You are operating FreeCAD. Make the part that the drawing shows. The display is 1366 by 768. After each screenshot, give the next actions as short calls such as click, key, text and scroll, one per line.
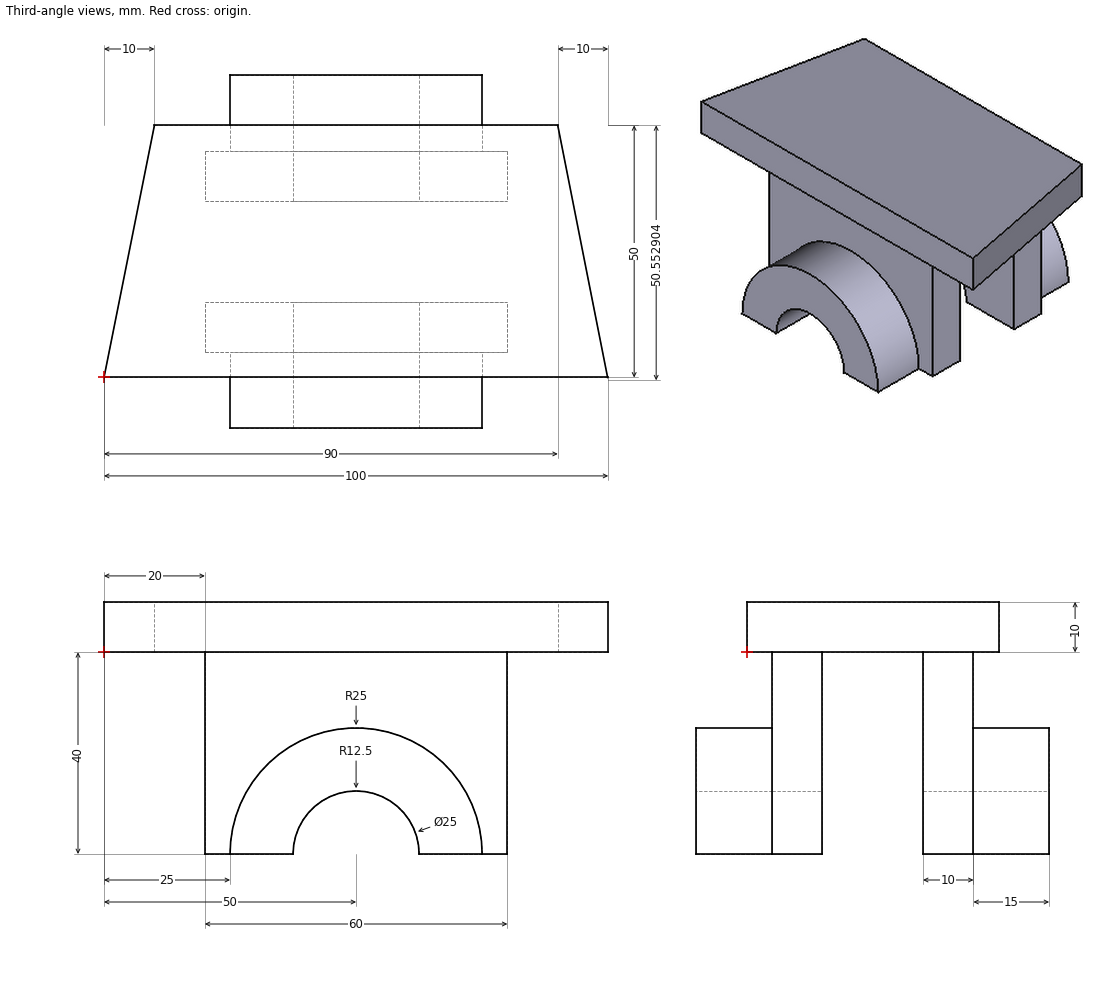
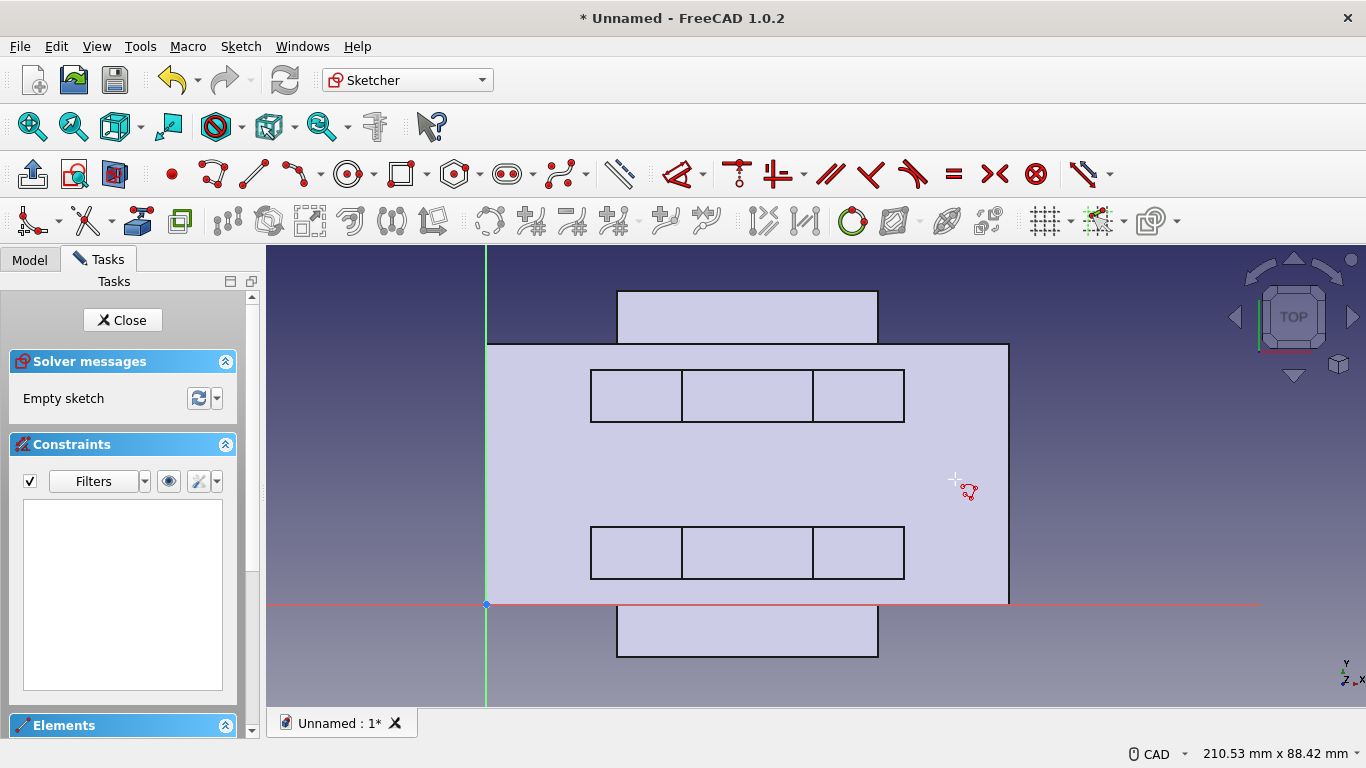
scroll(1009, 608, up, 9)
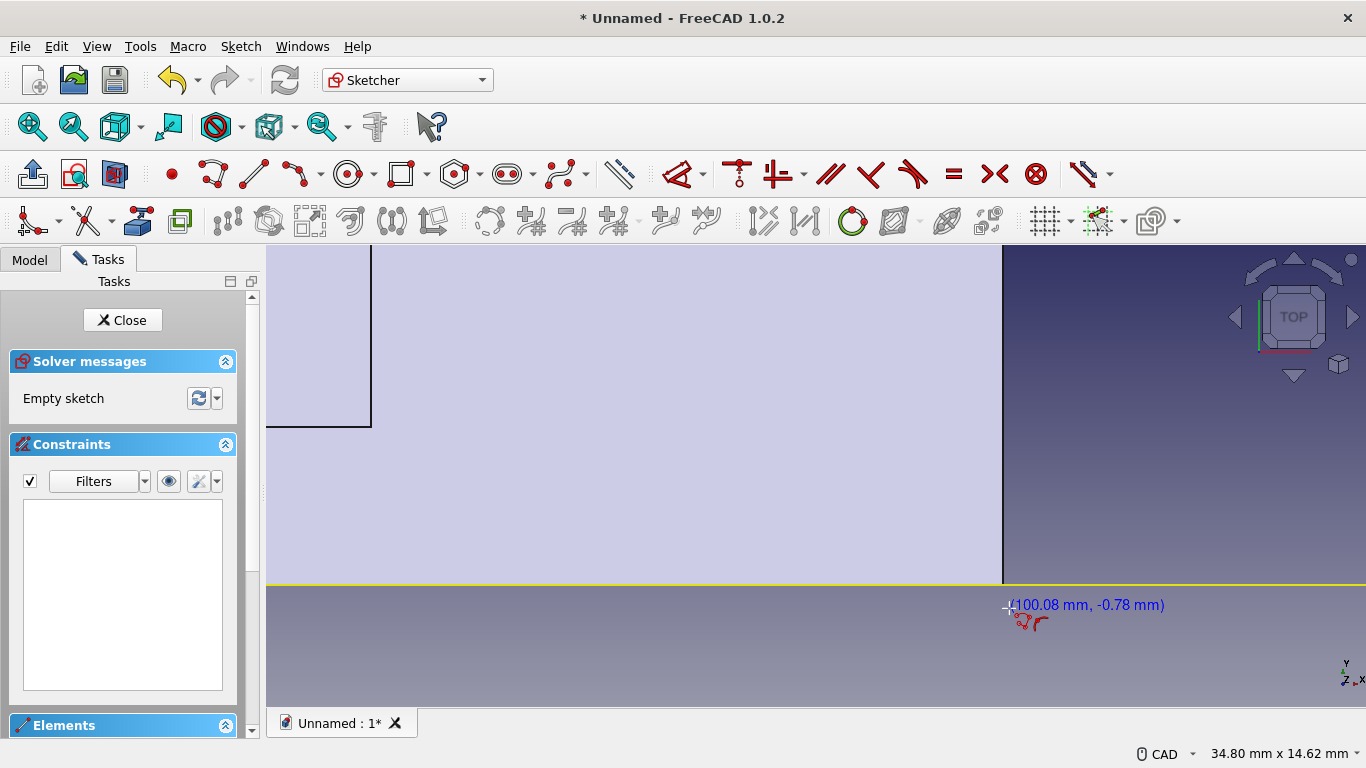
click(1003, 603)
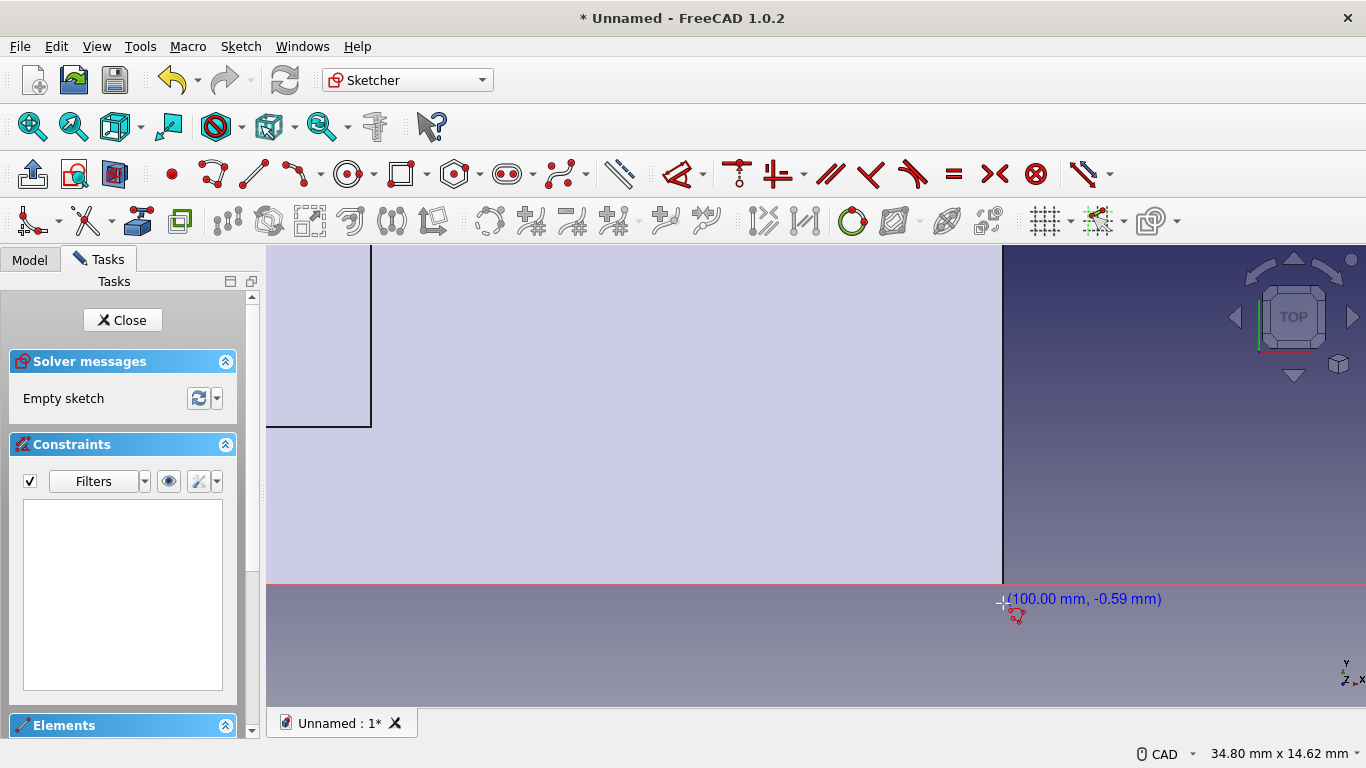
scroll(1010, 609, down, 9)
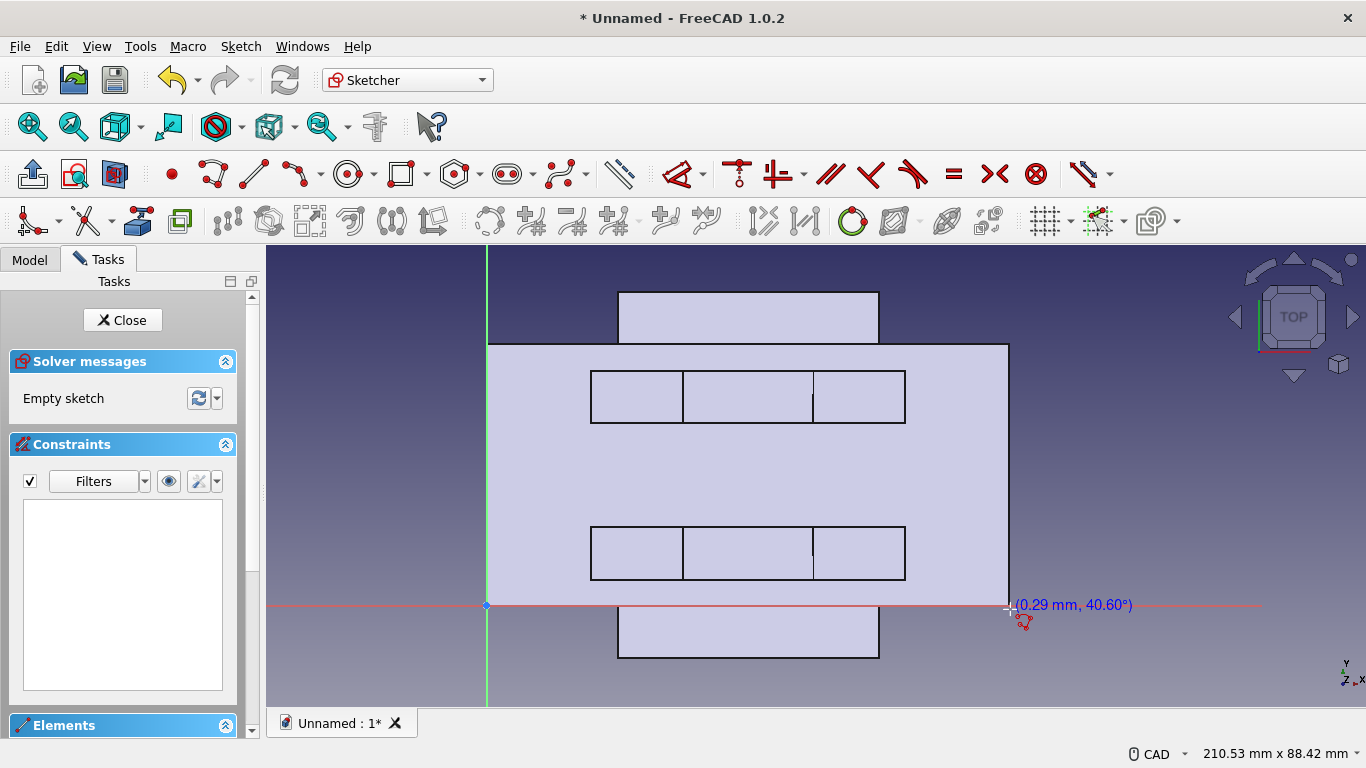
click(957, 344)
click(1009, 344)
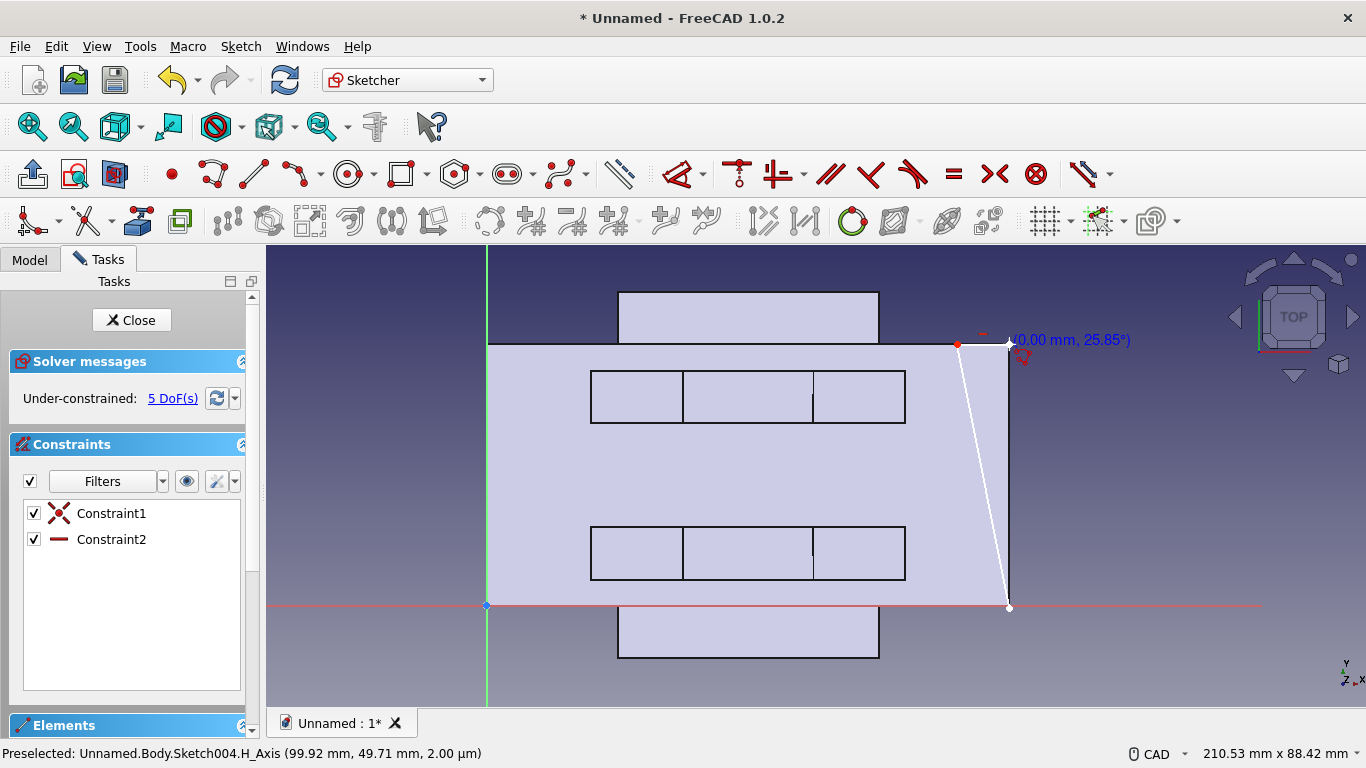
scroll(1009, 609, up, 9)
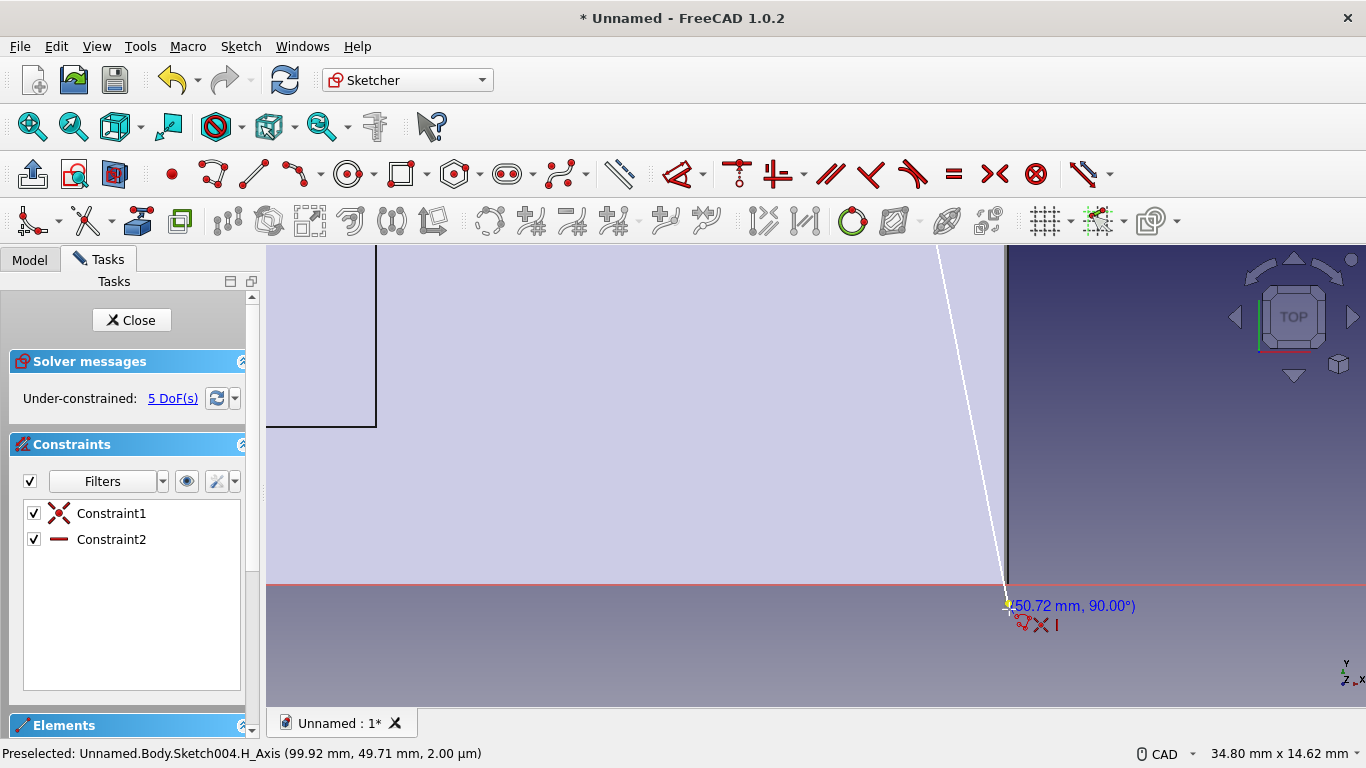
click(1008, 604)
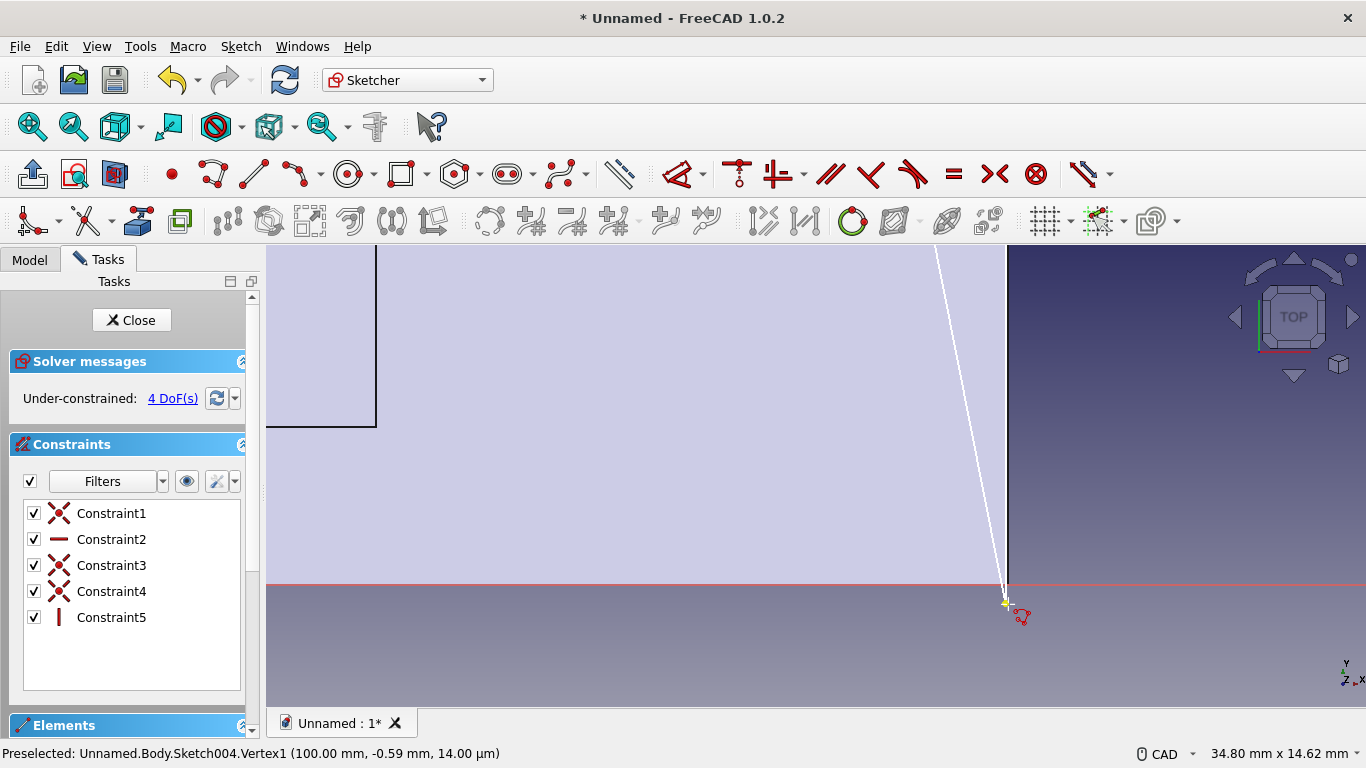
scroll(1009, 609, down, 9)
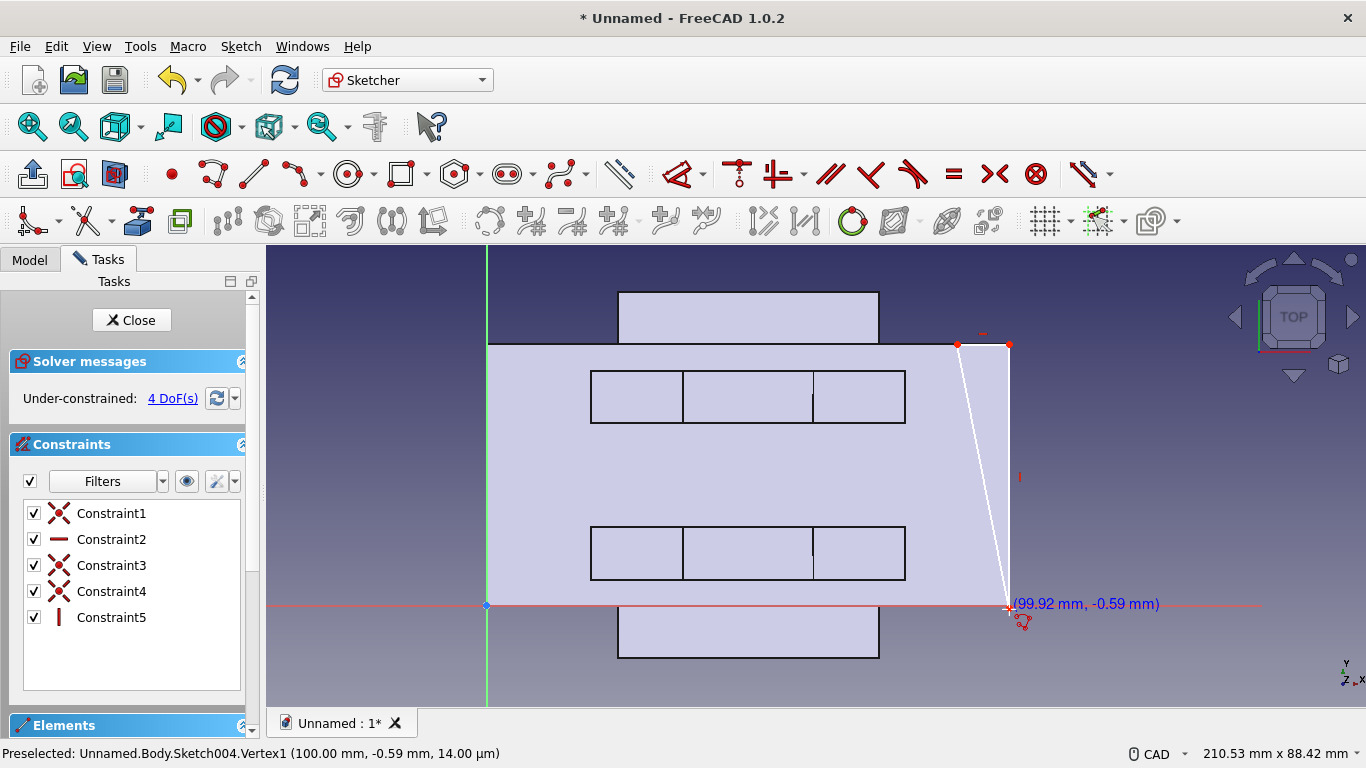
click(487, 606)
click(496, 344)
click(539, 344)
click(487, 606)
key(Escape)
key(Escape)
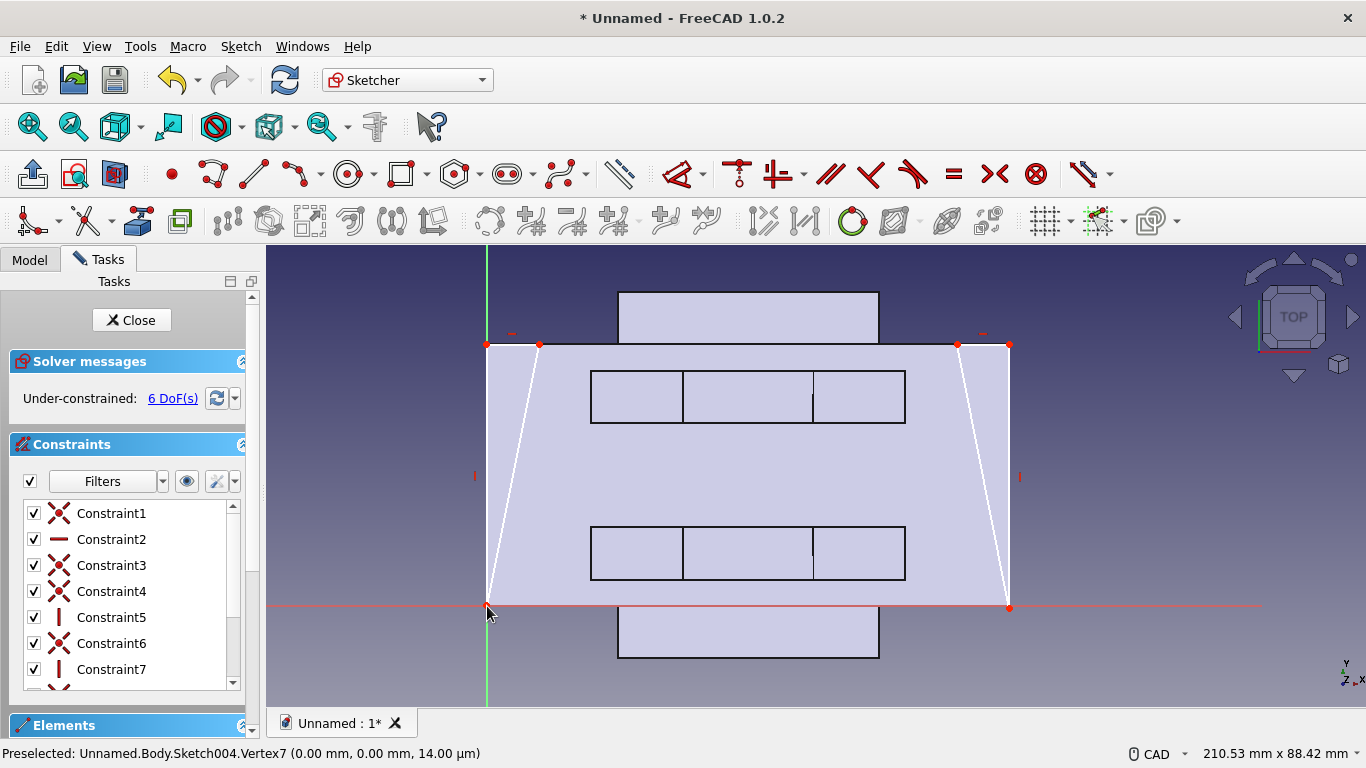
click(676, 174)